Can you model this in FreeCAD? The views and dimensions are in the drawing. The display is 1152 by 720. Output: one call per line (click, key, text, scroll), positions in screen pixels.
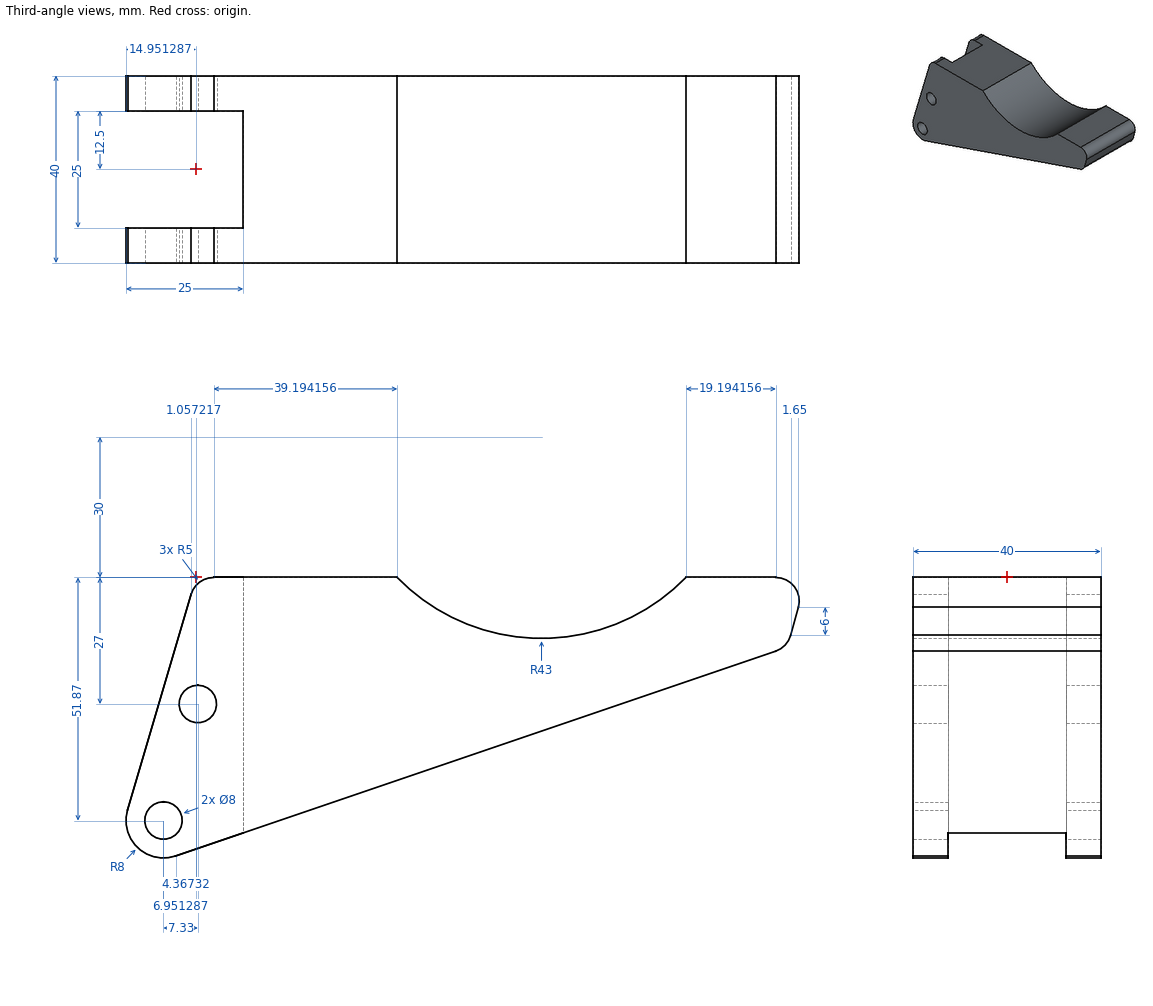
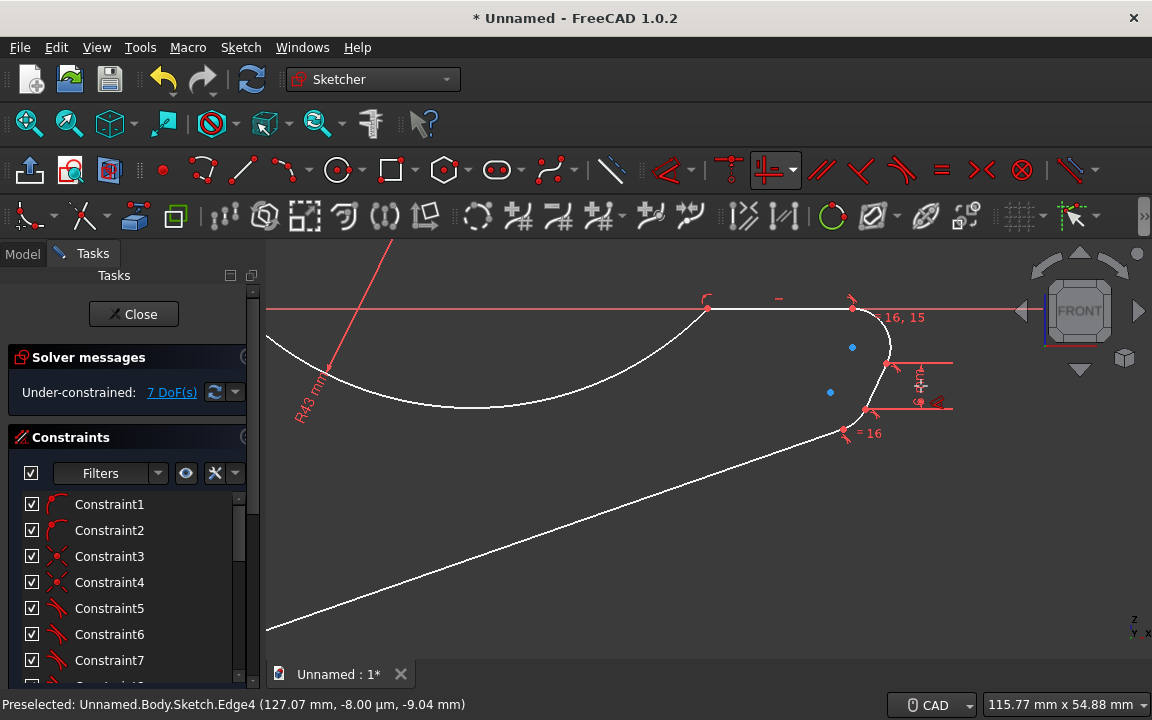
scroll(883, 378, down, 4)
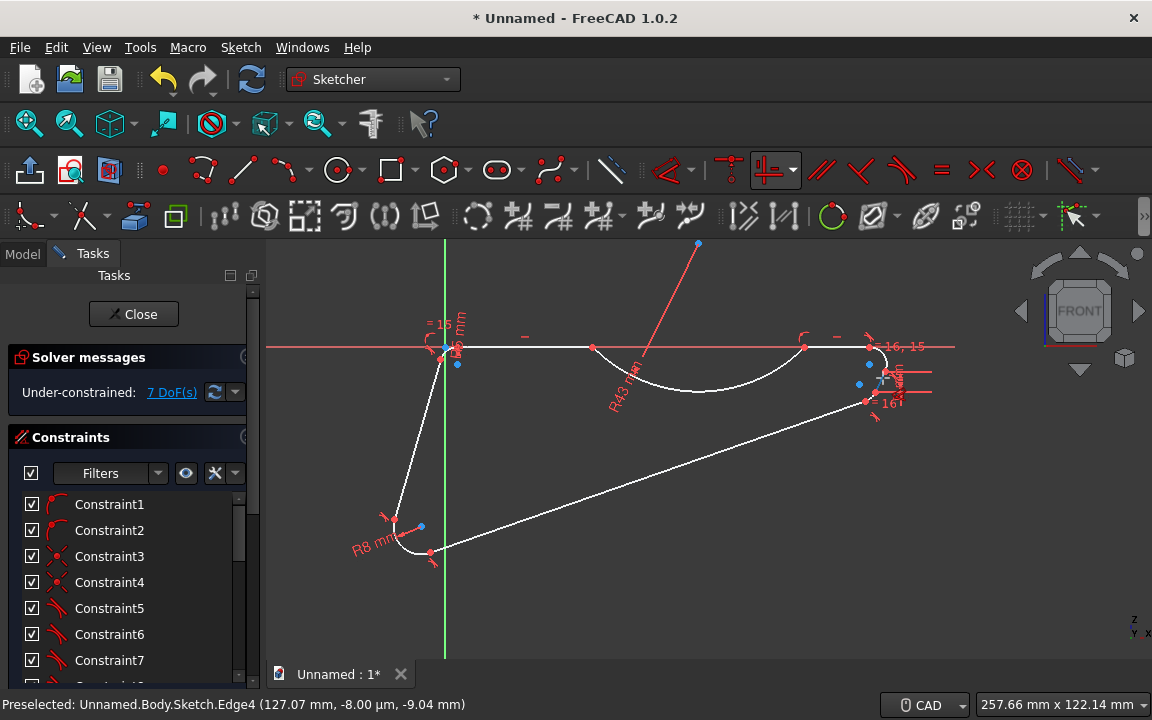
scroll(639, 631, down, 1)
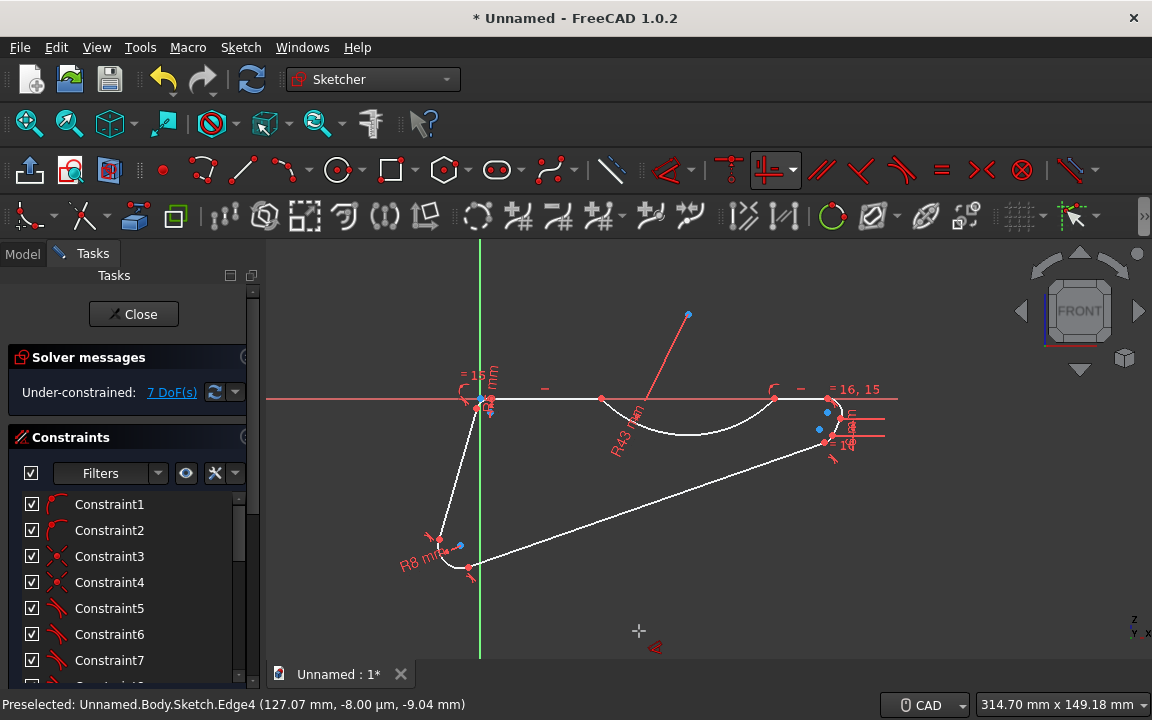
click(688, 314)
click(446, 356)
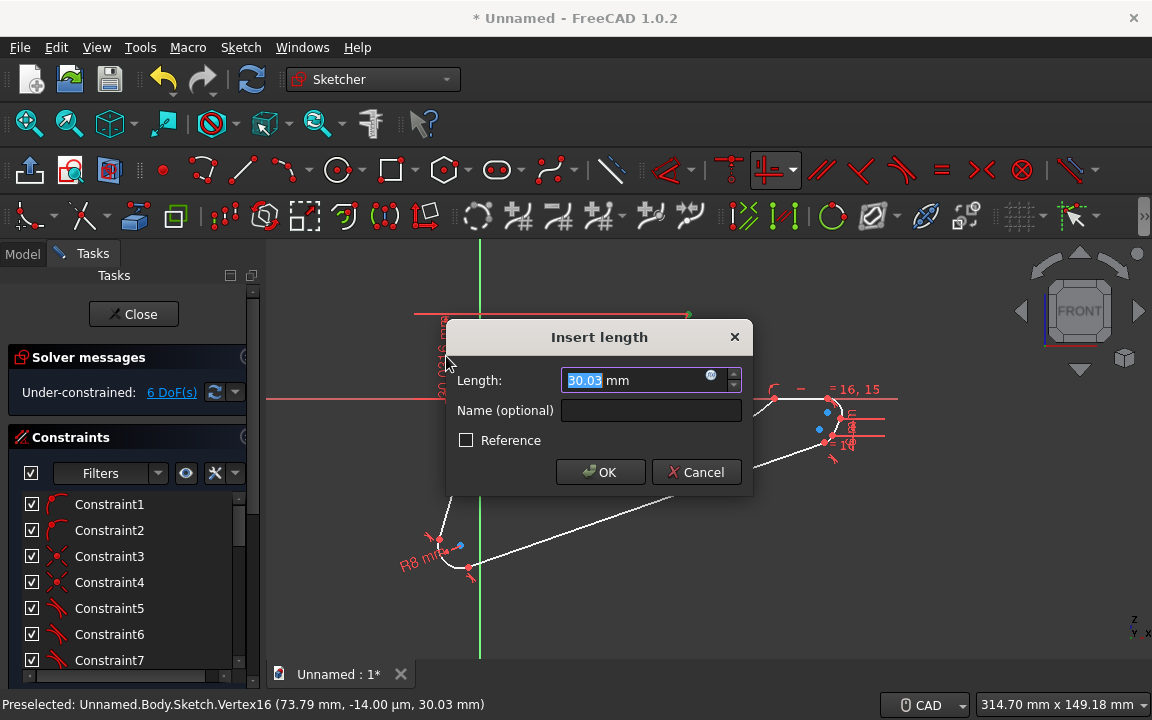
text(30)
key(Return)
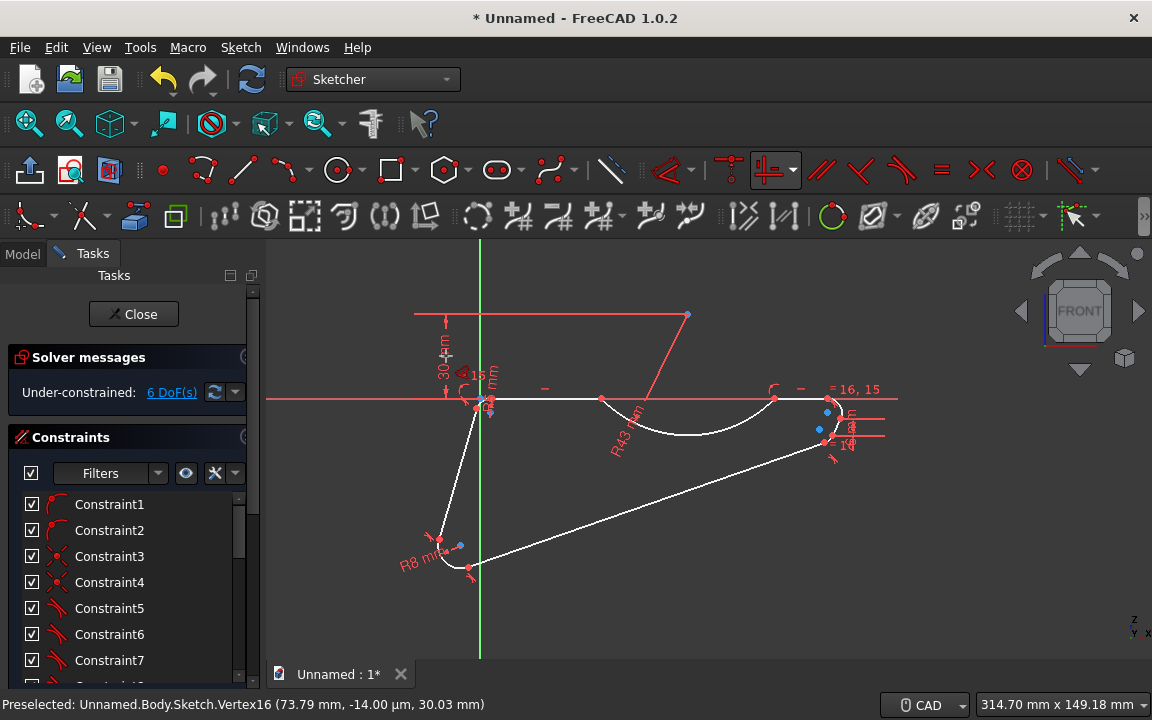
scroll(837, 427, up, 11)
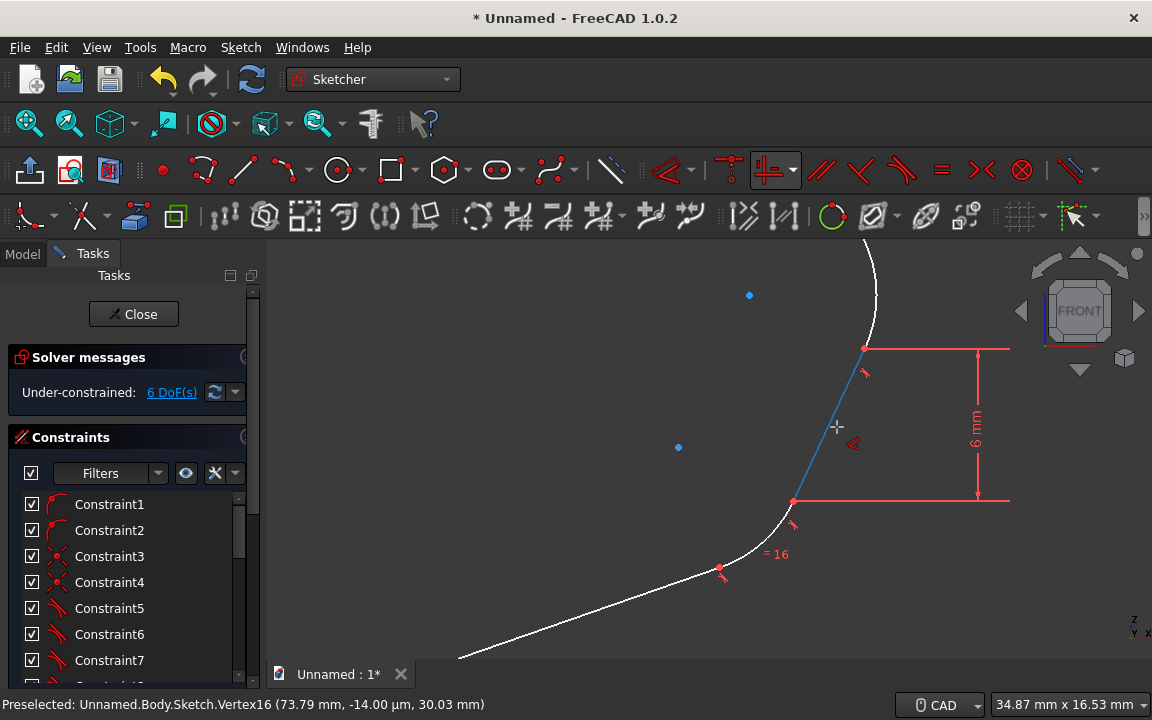
click(829, 425)
click(829, 315)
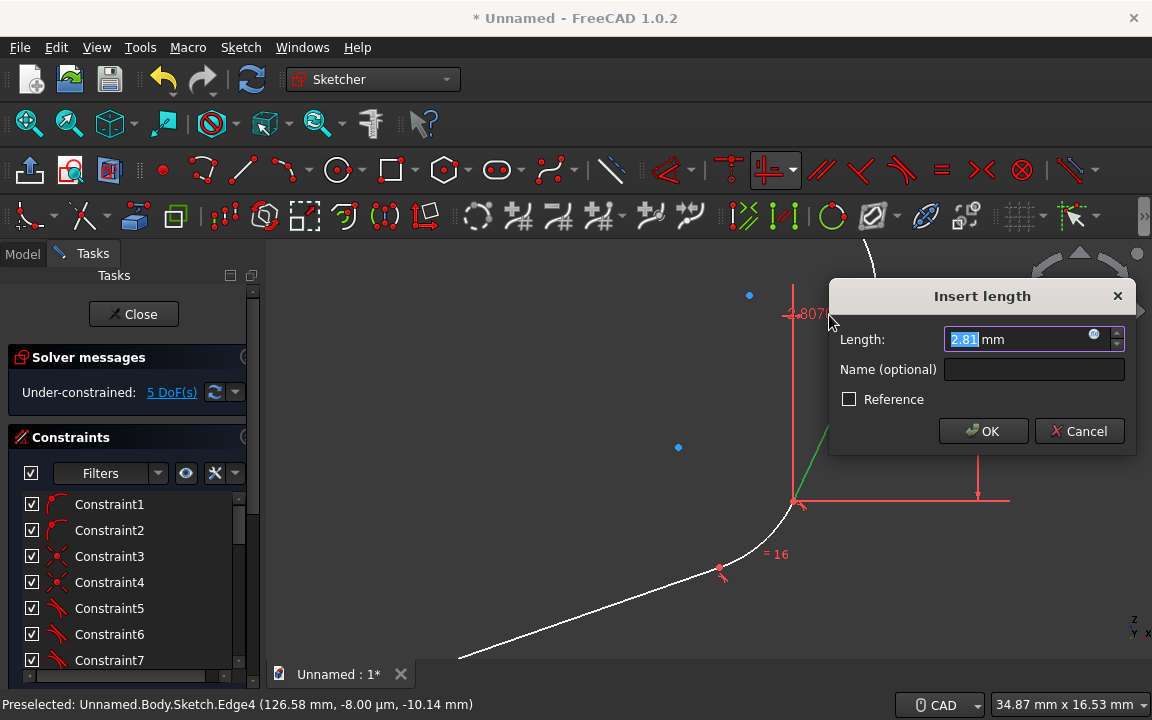
text(1.65)
key(Return)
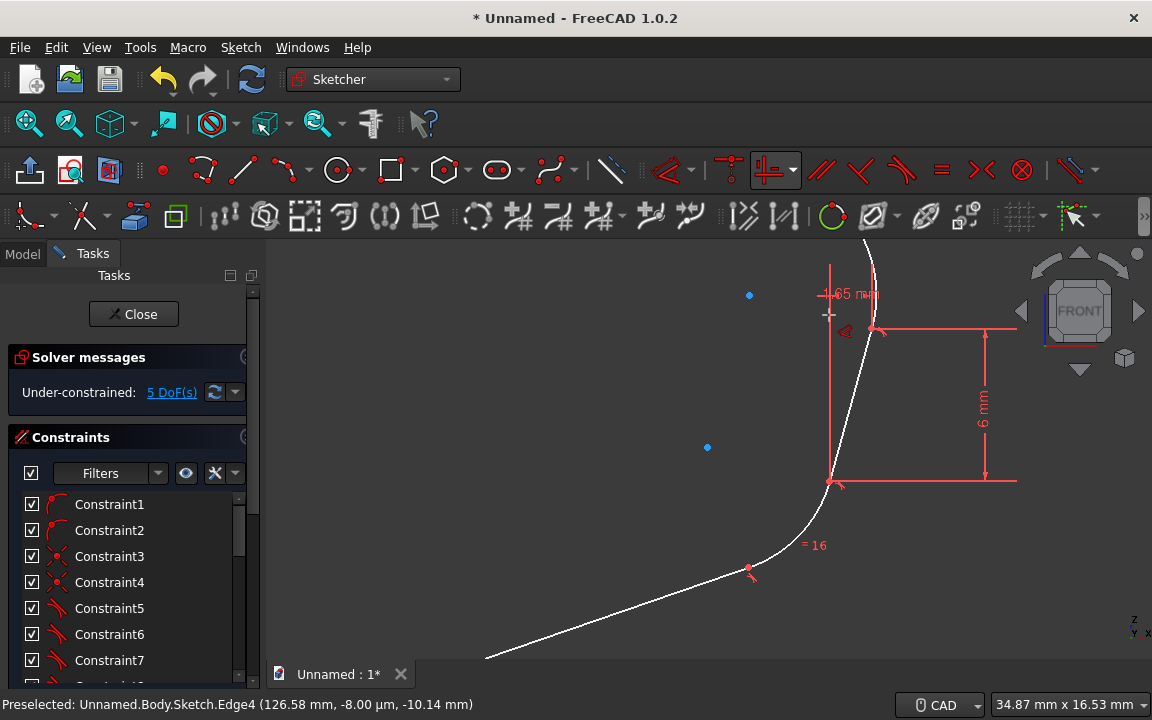
scroll(888, 375, down, 10)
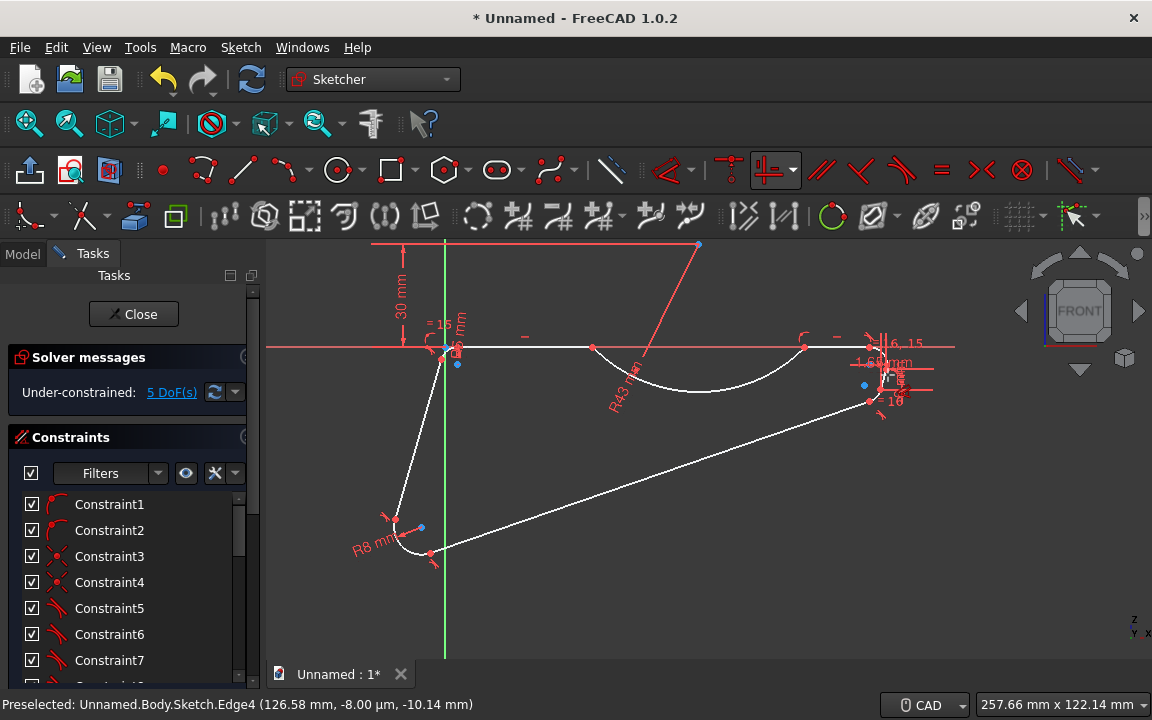
click(422, 527)
click(388, 437)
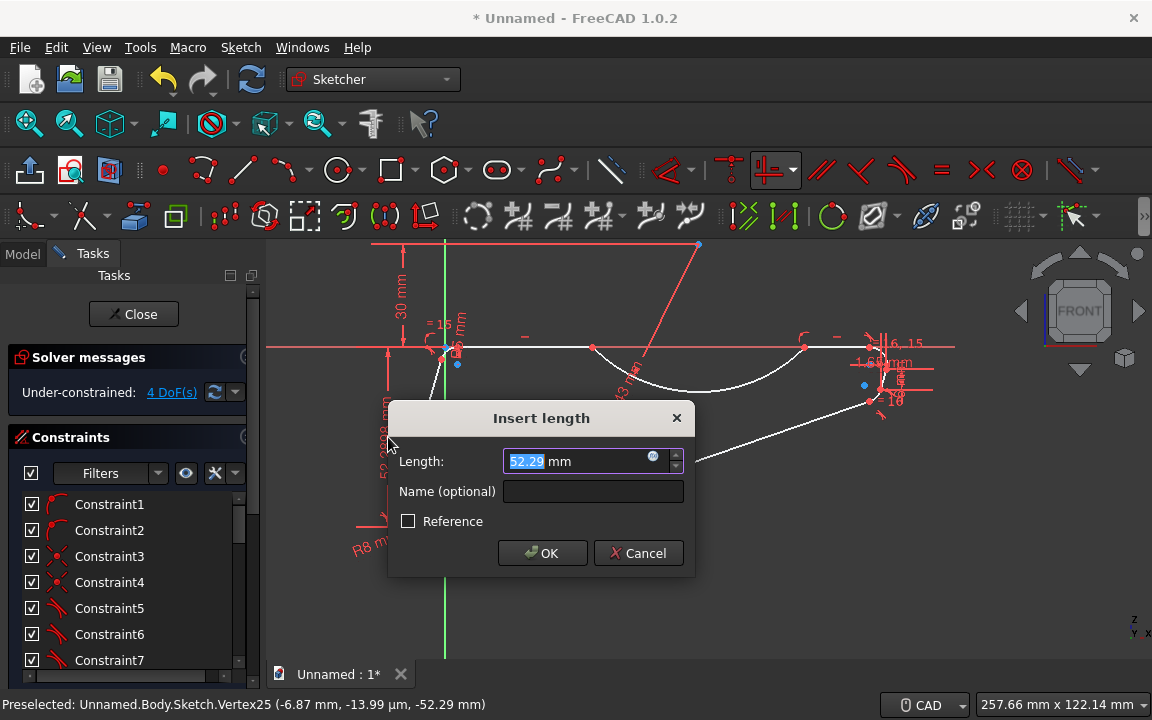
text(51.87)
key(Return)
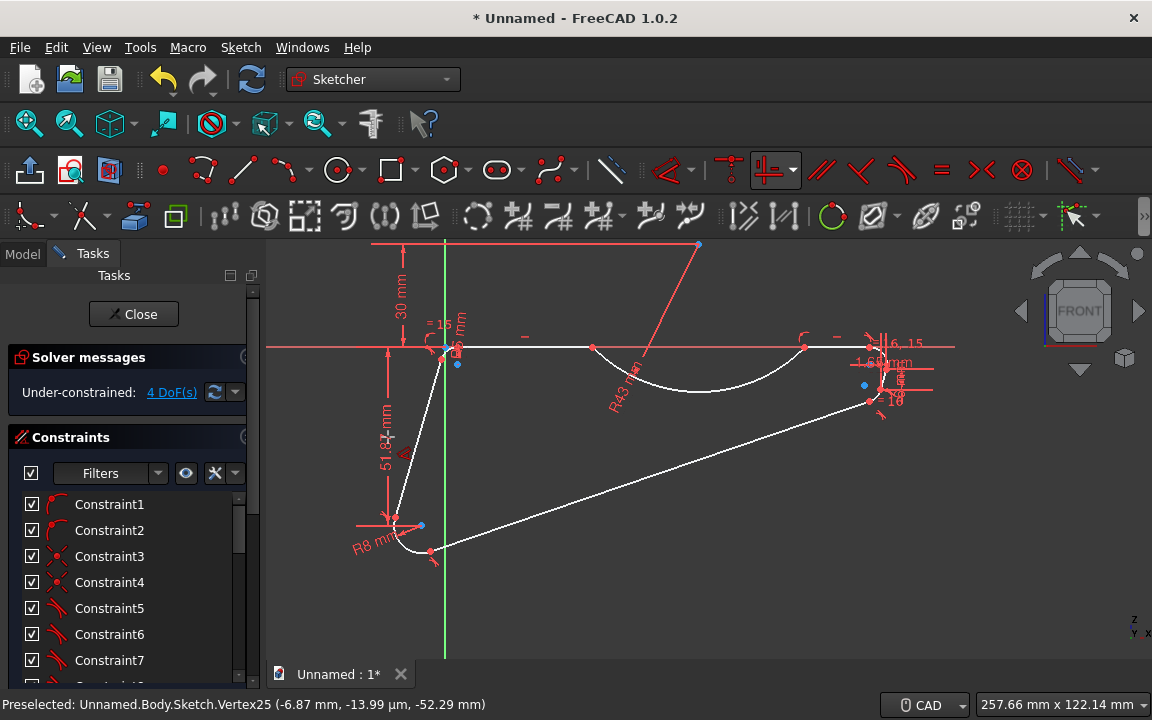
scroll(431, 552, up, 5)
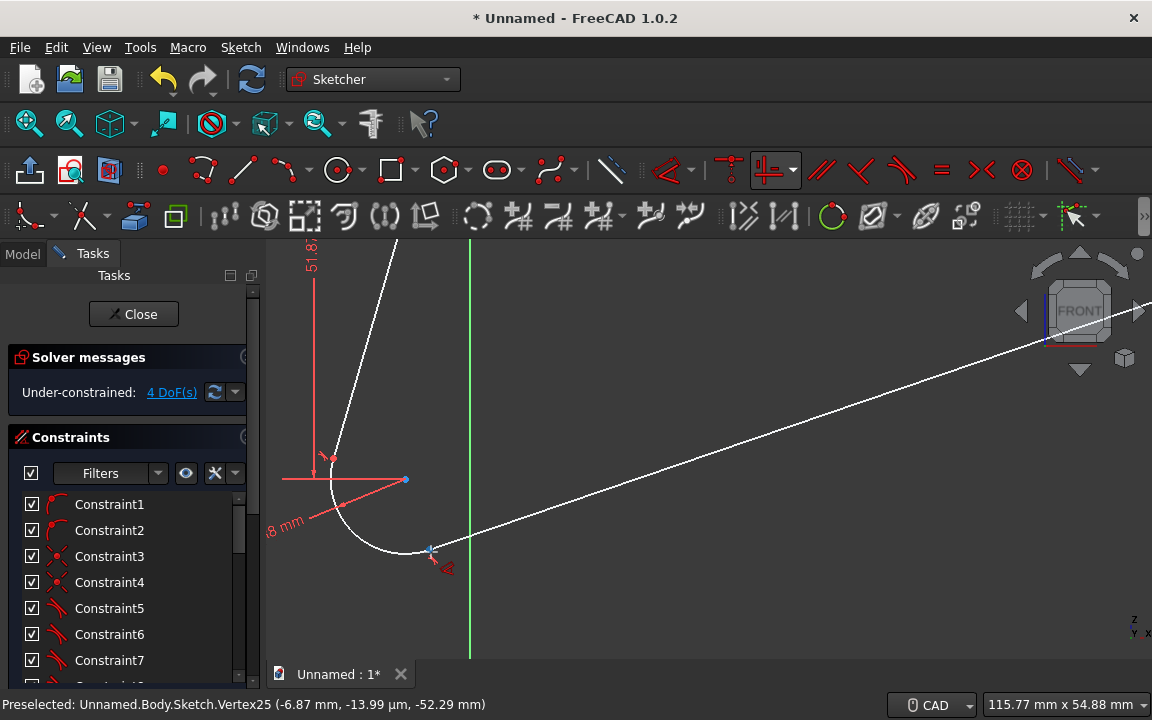
click(430, 550)
click(450, 584)